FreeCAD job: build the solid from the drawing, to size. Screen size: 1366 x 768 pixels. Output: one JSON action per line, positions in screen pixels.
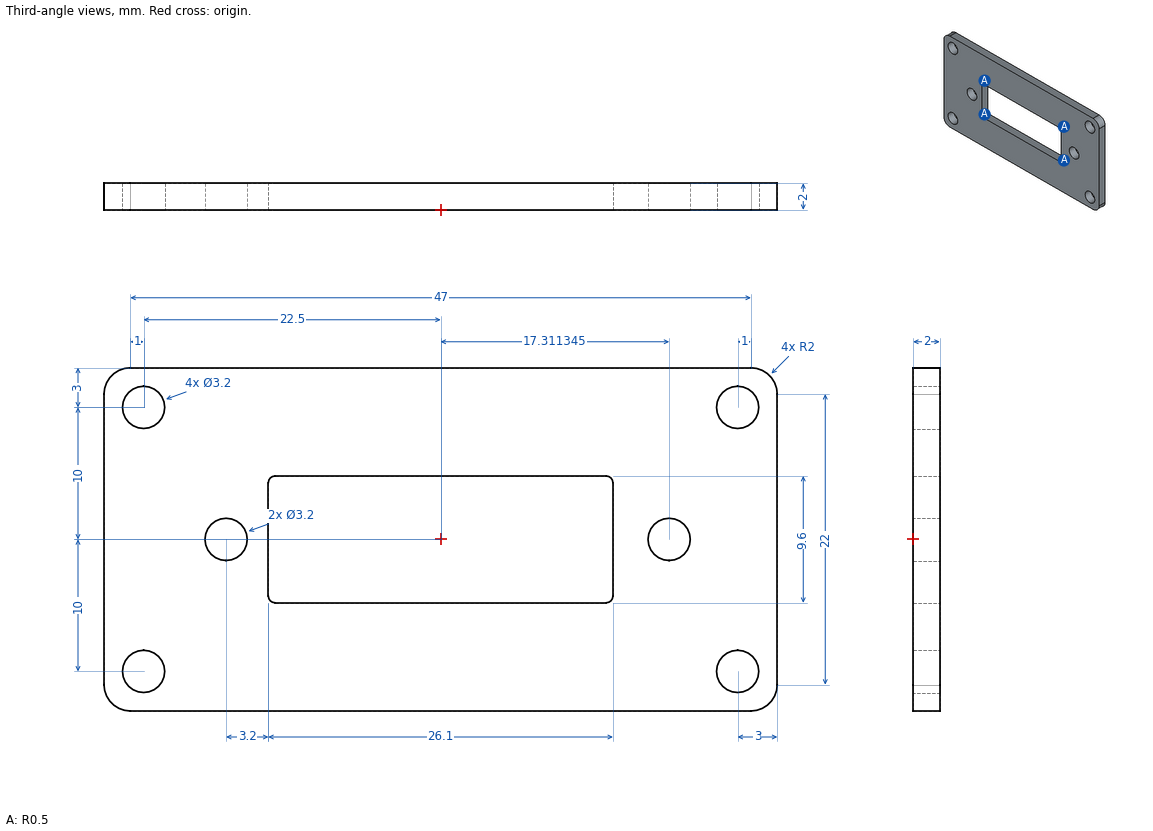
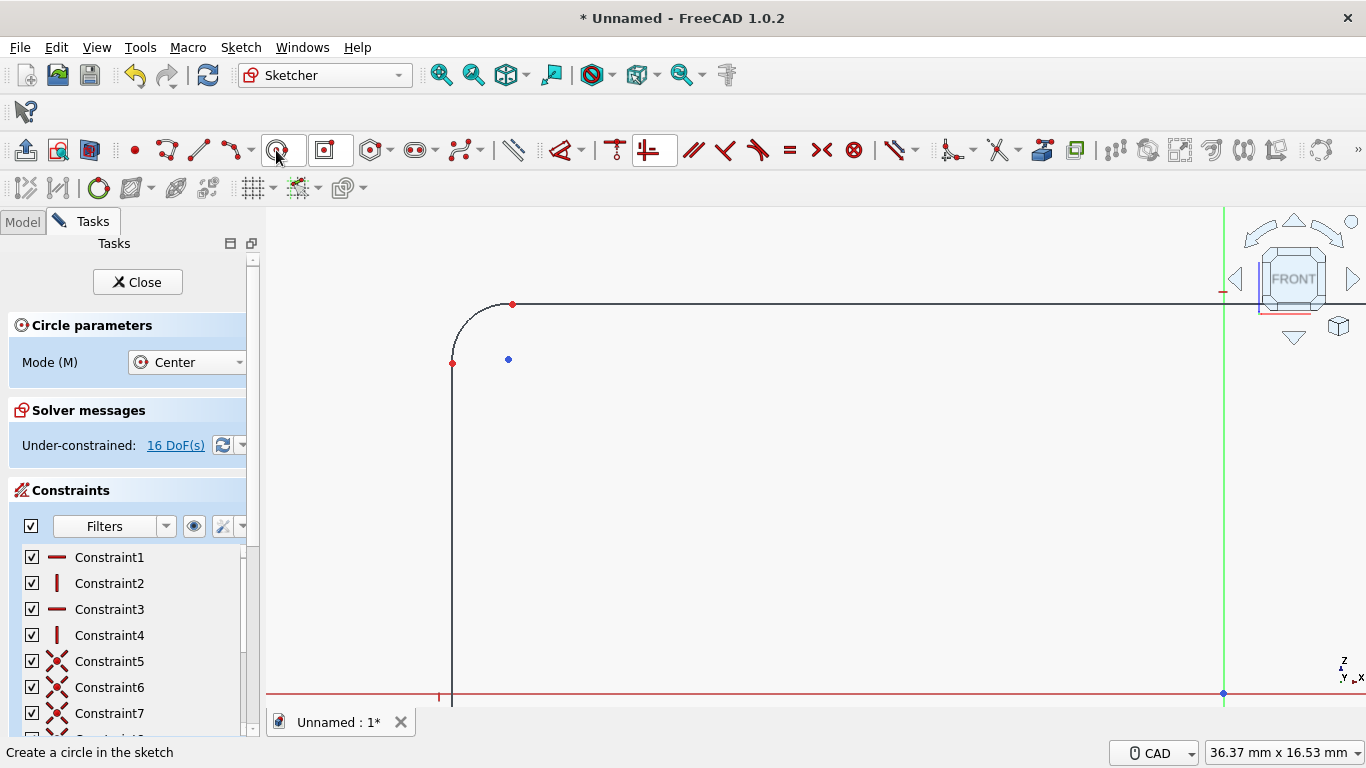
{"action": "left_click", "coordinate": [543, 391]}
{"action": "left_click", "coordinate": [577, 357]}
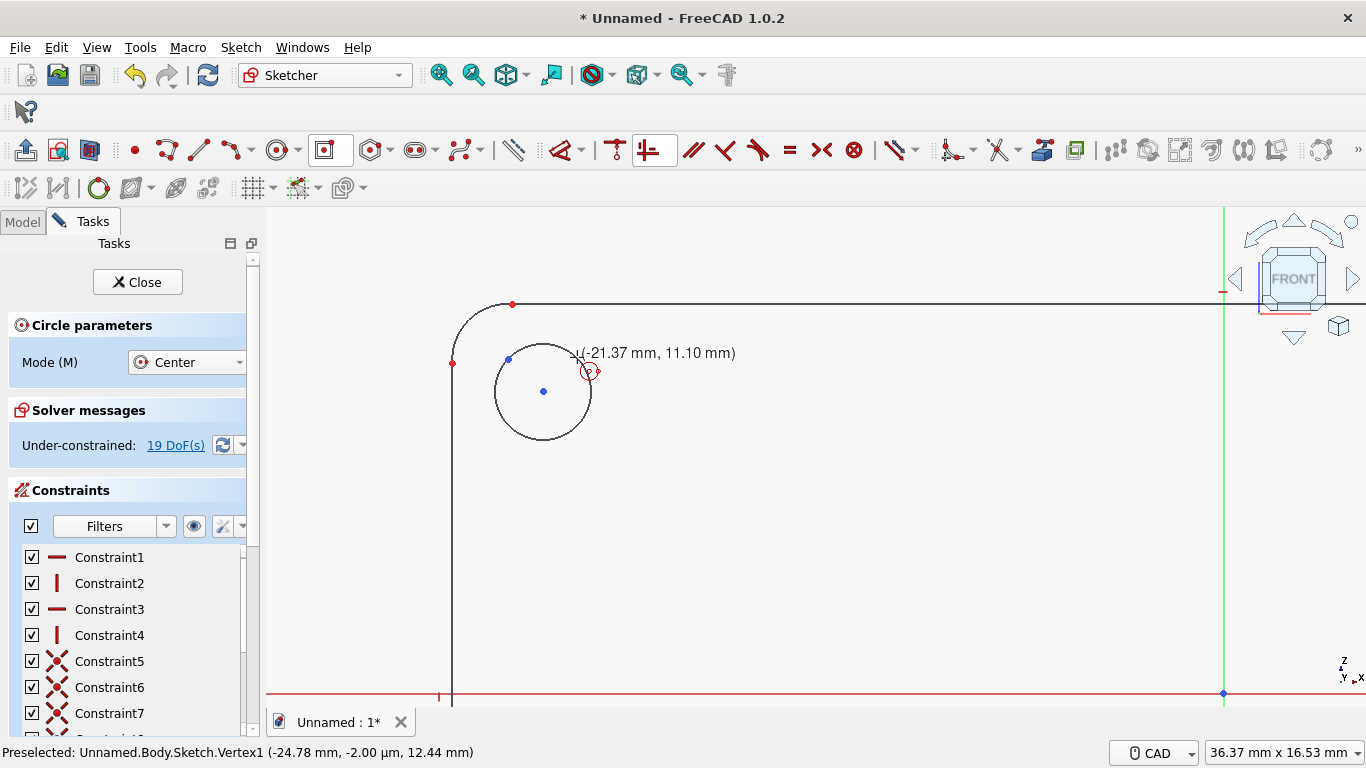
{"action": "scroll", "coordinate": [470, 319], "scroll_direction": "down", "scroll_amount": 5}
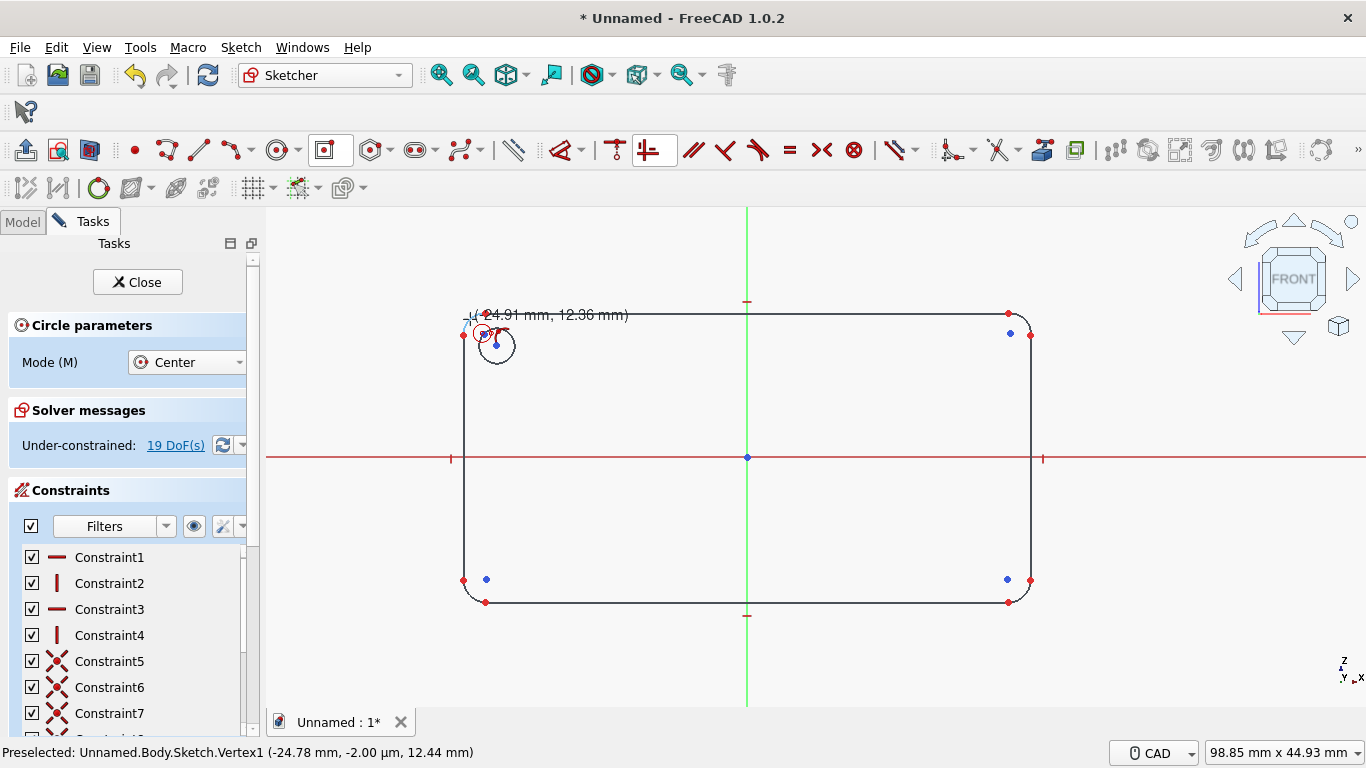
{"action": "scroll", "coordinate": [998, 346], "scroll_direction": "up", "scroll_amount": 2}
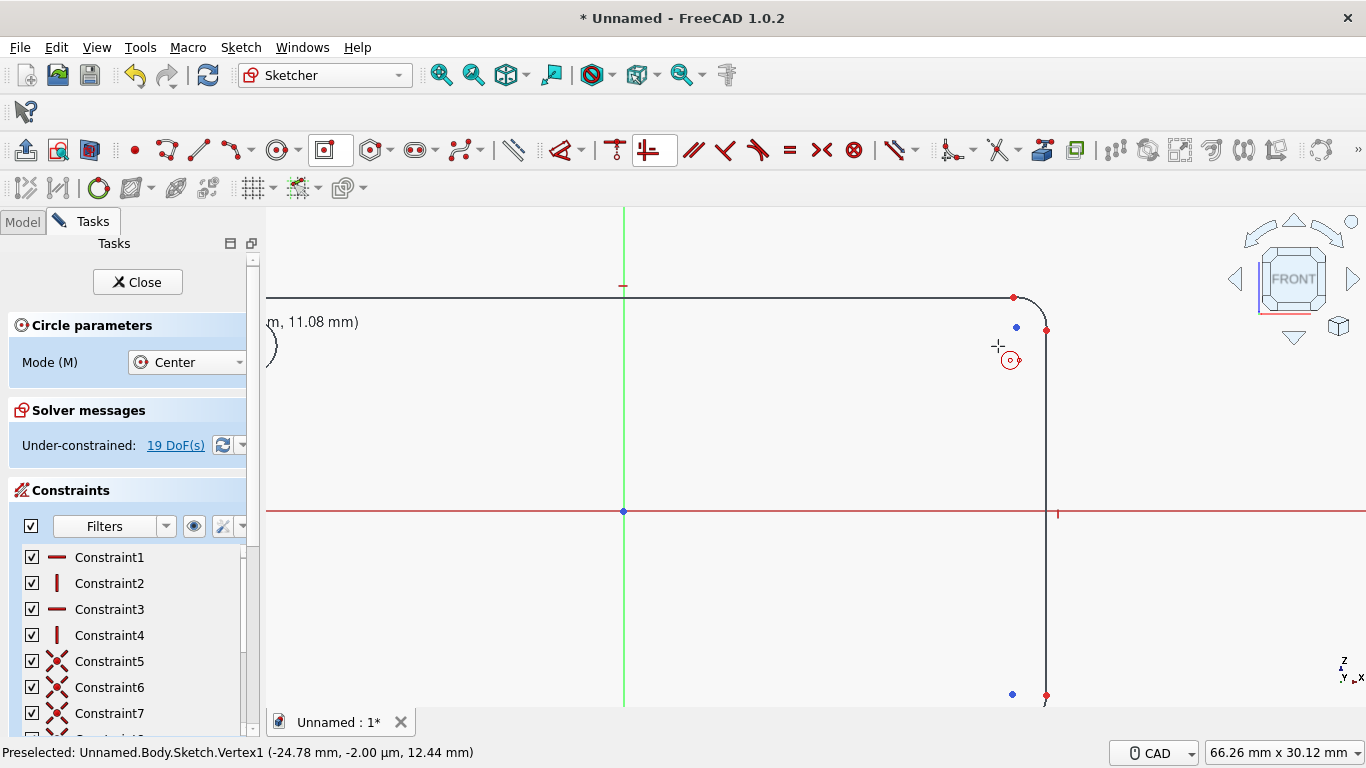
{"action": "left_click", "coordinate": [997, 345]}
{"action": "left_click", "coordinate": [978, 327]}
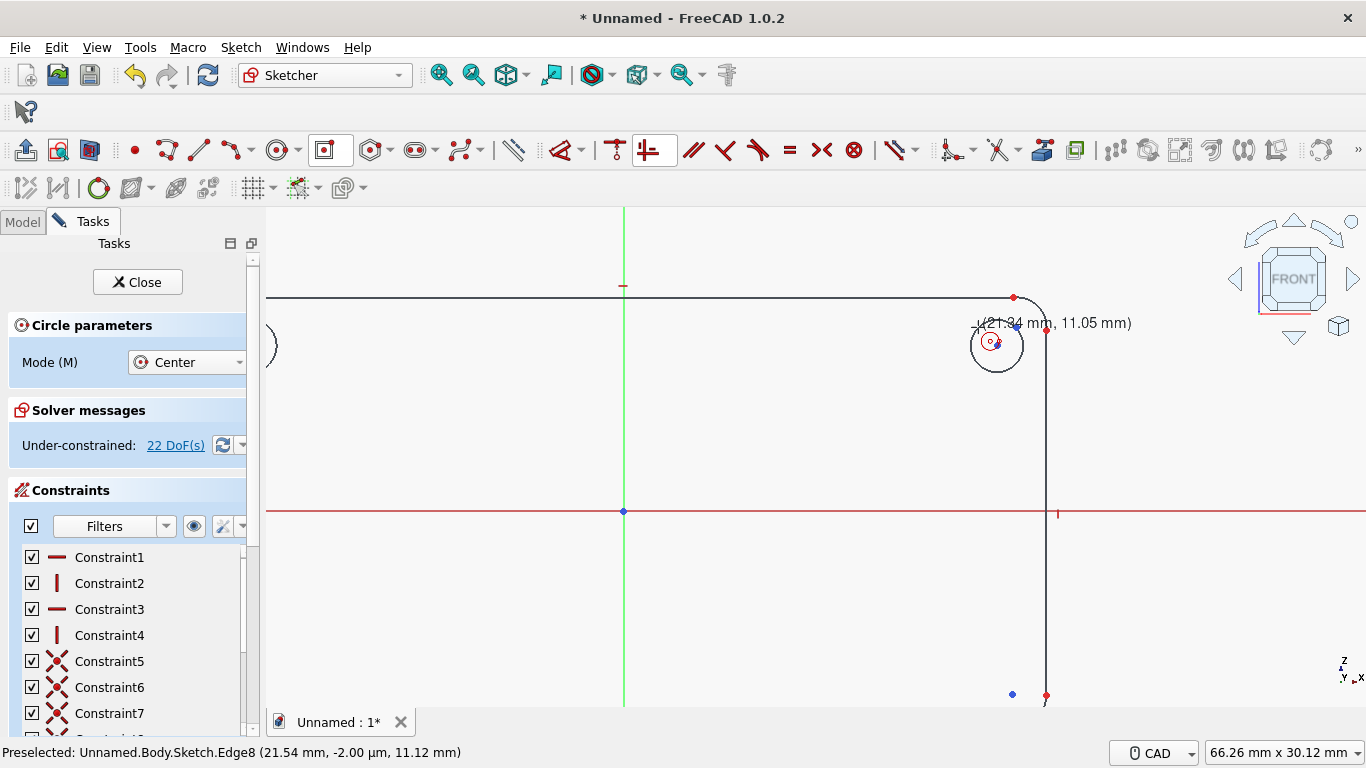
{"action": "scroll", "coordinate": [999, 346], "scroll_direction": "down", "scroll_amount": 2}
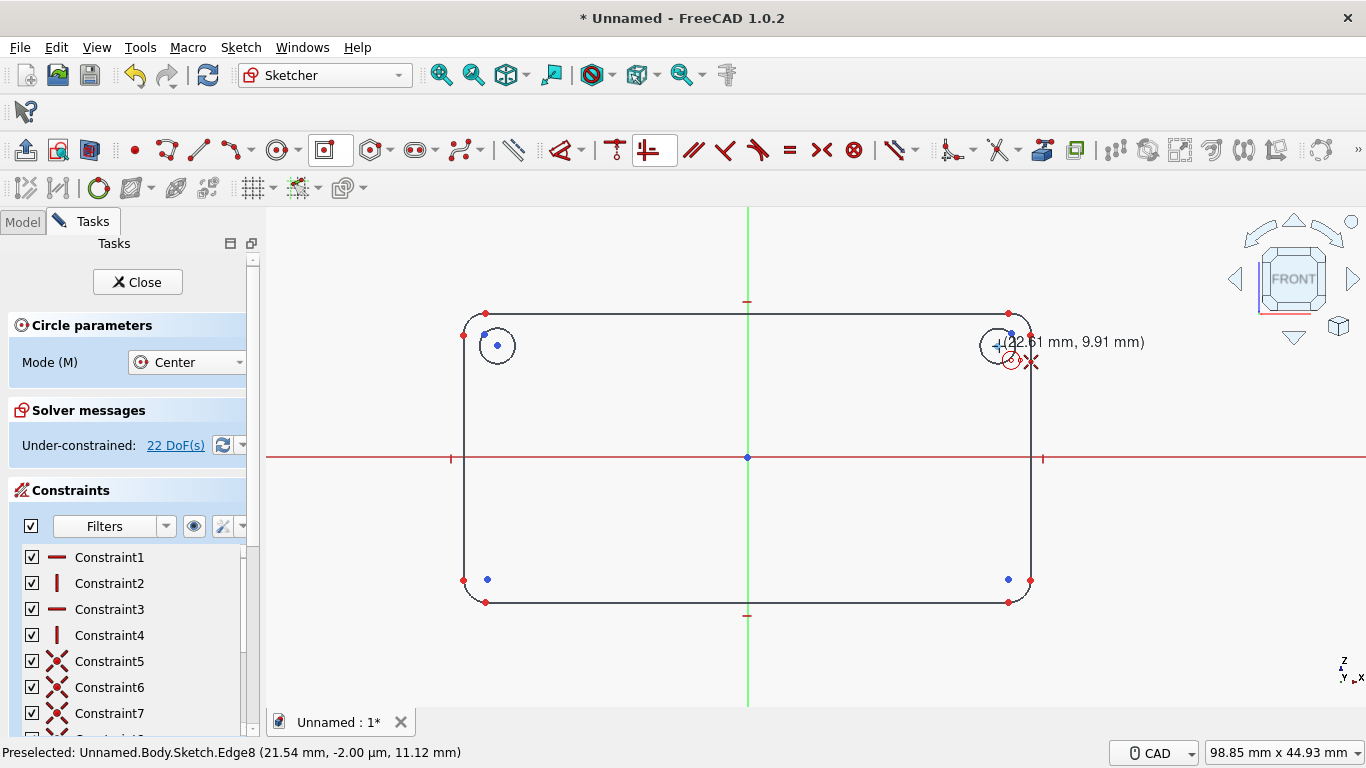
{"action": "scroll", "coordinate": [497, 568], "scroll_direction": "up", "scroll_amount": 2}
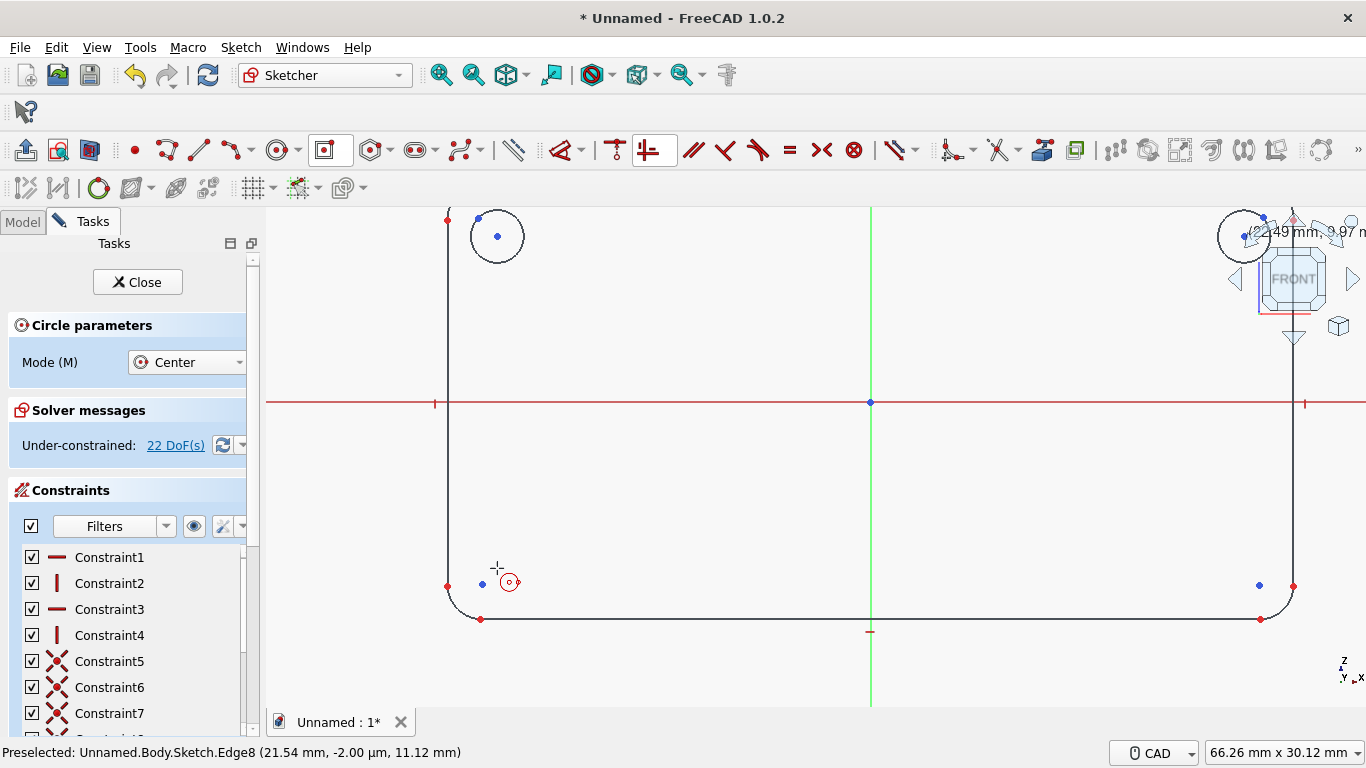
{"action": "left_click", "coordinate": [497, 568]}
{"action": "left_click", "coordinate": [516, 549]}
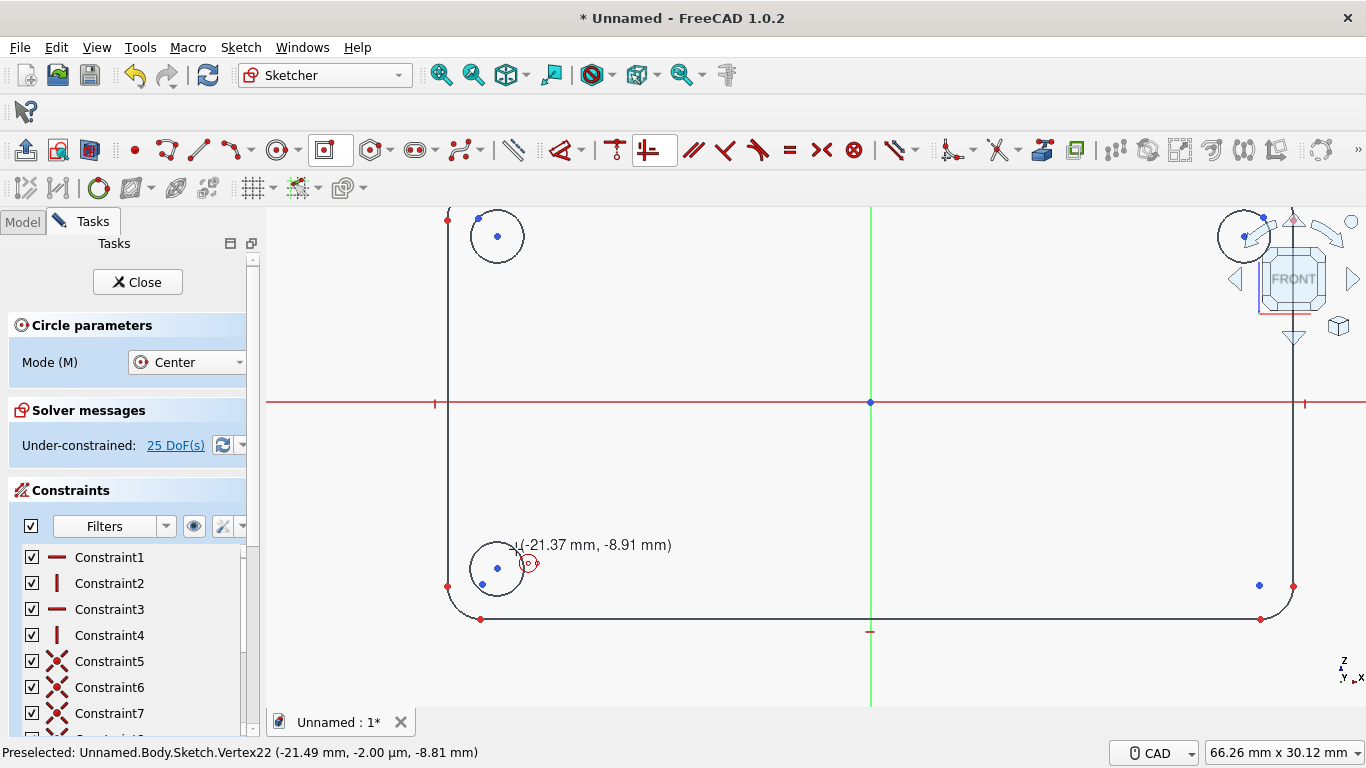
{"action": "scroll", "coordinate": [497, 569], "scroll_direction": "down", "scroll_amount": 2}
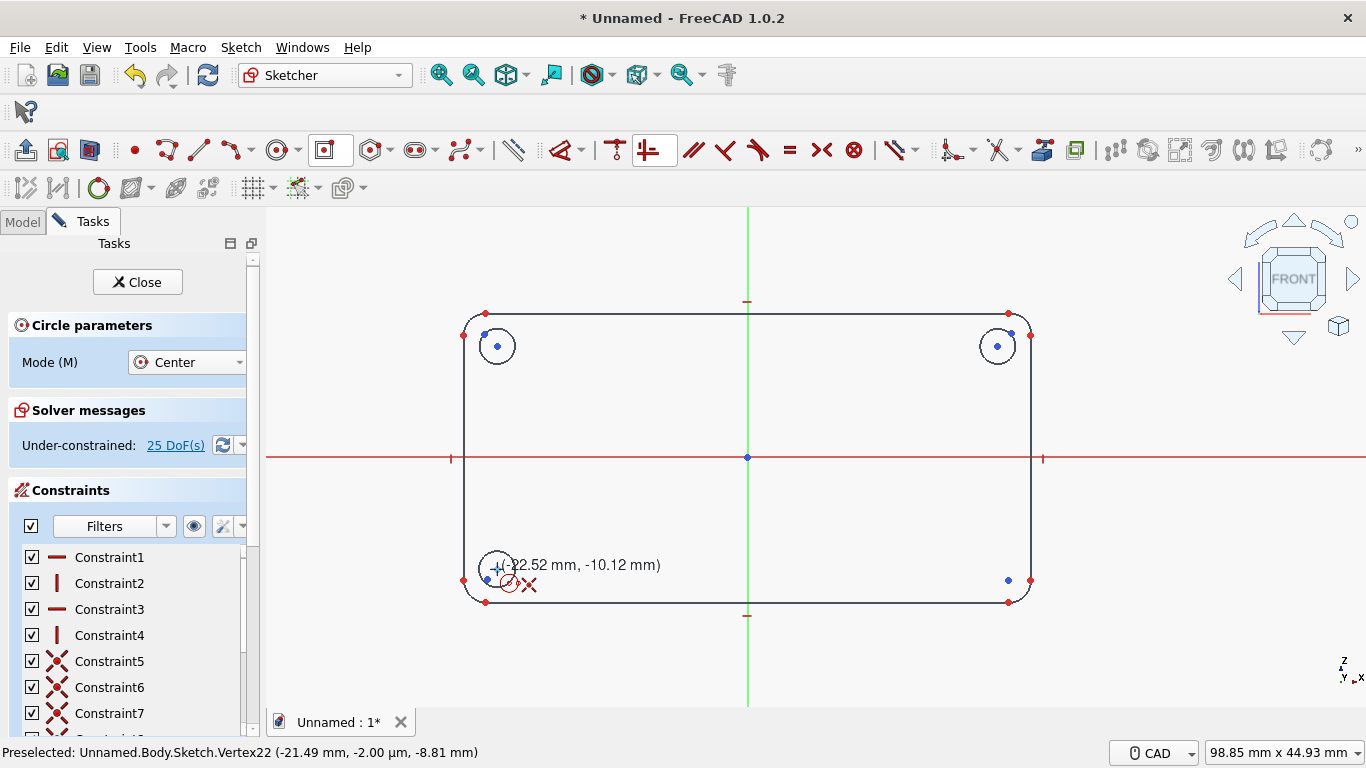
{"action": "scroll", "coordinate": [998, 569], "scroll_direction": "up", "scroll_amount": 2}